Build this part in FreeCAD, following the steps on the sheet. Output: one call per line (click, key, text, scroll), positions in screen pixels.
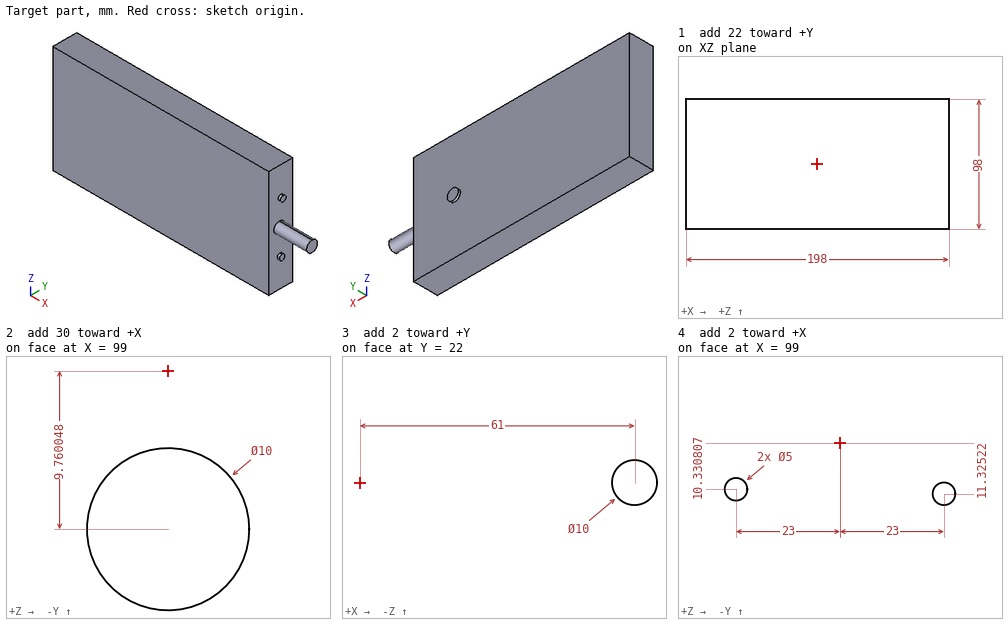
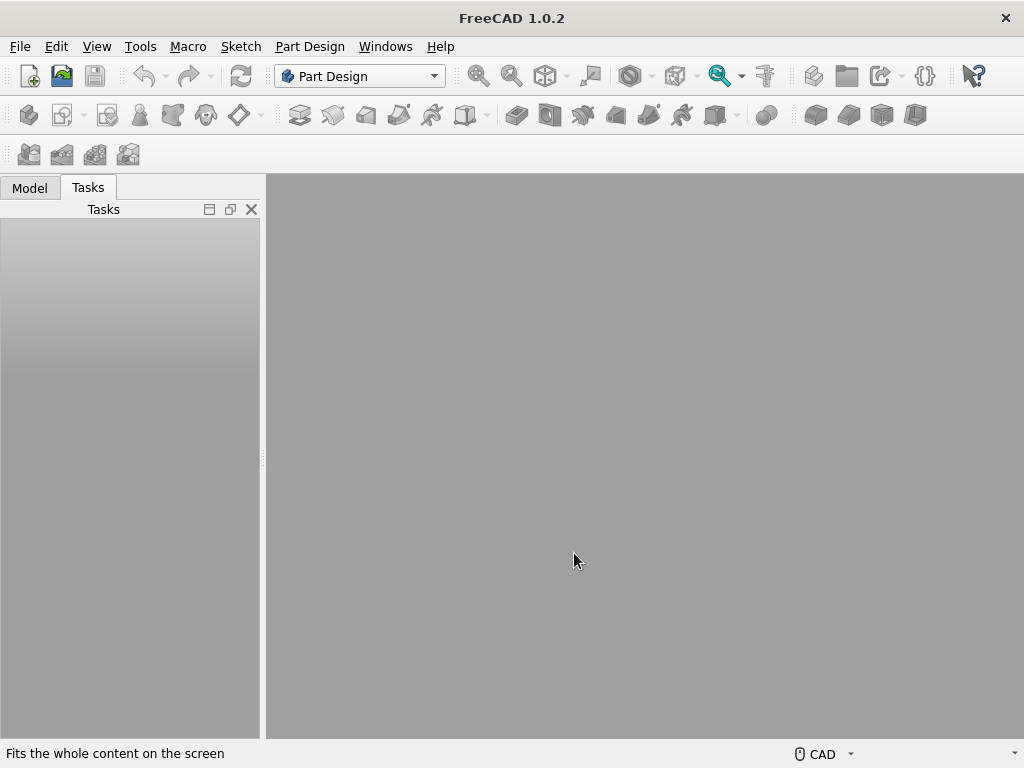
key(ctrl+n)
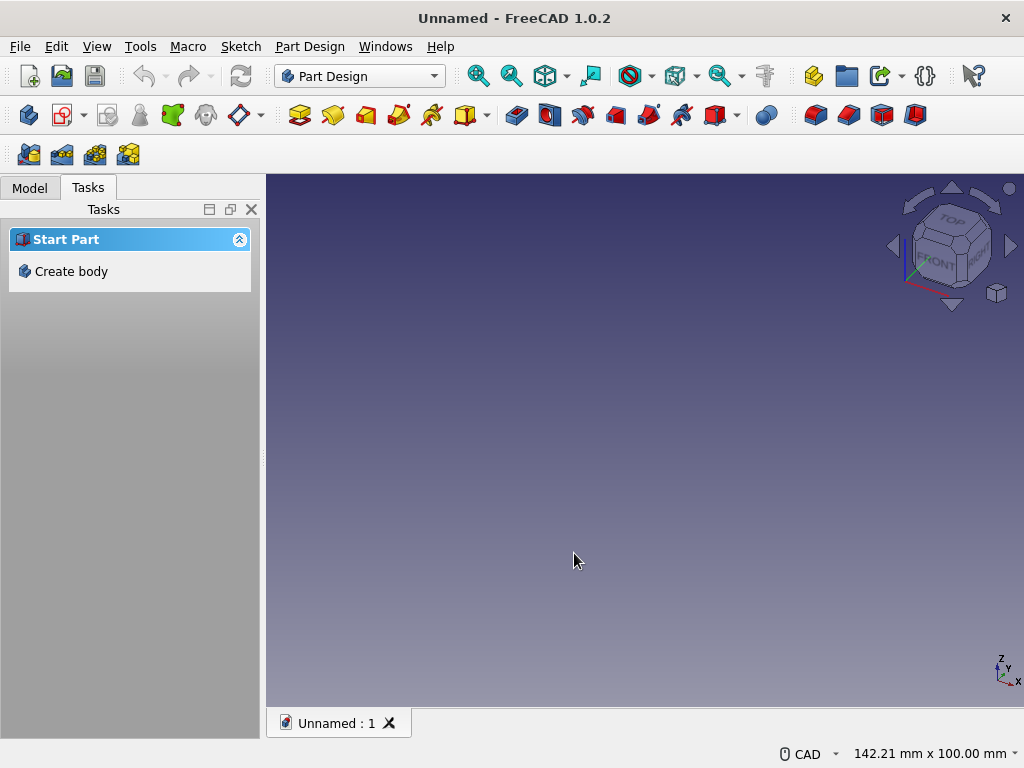
click(62, 116)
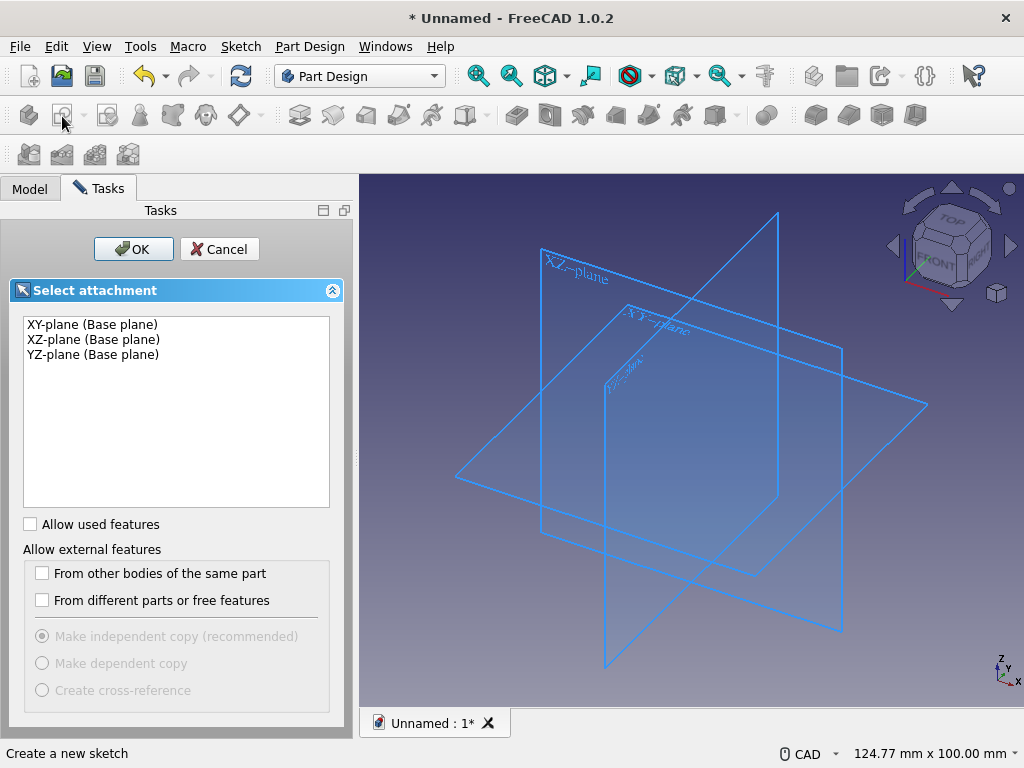
click(84, 340)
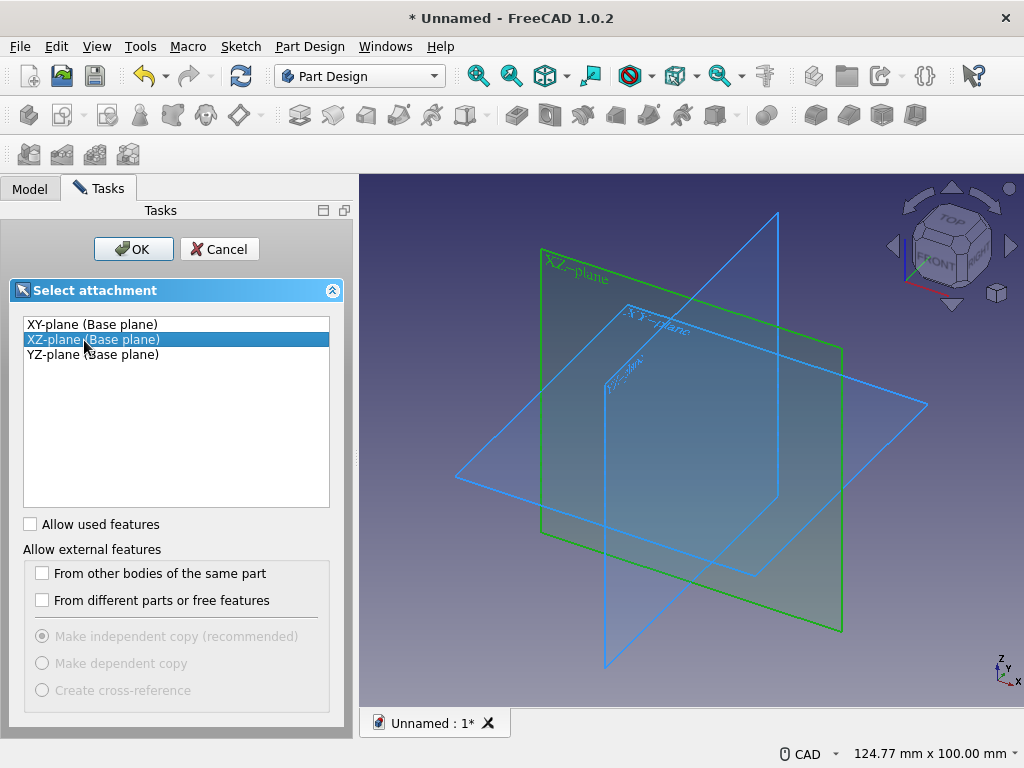
click(134, 249)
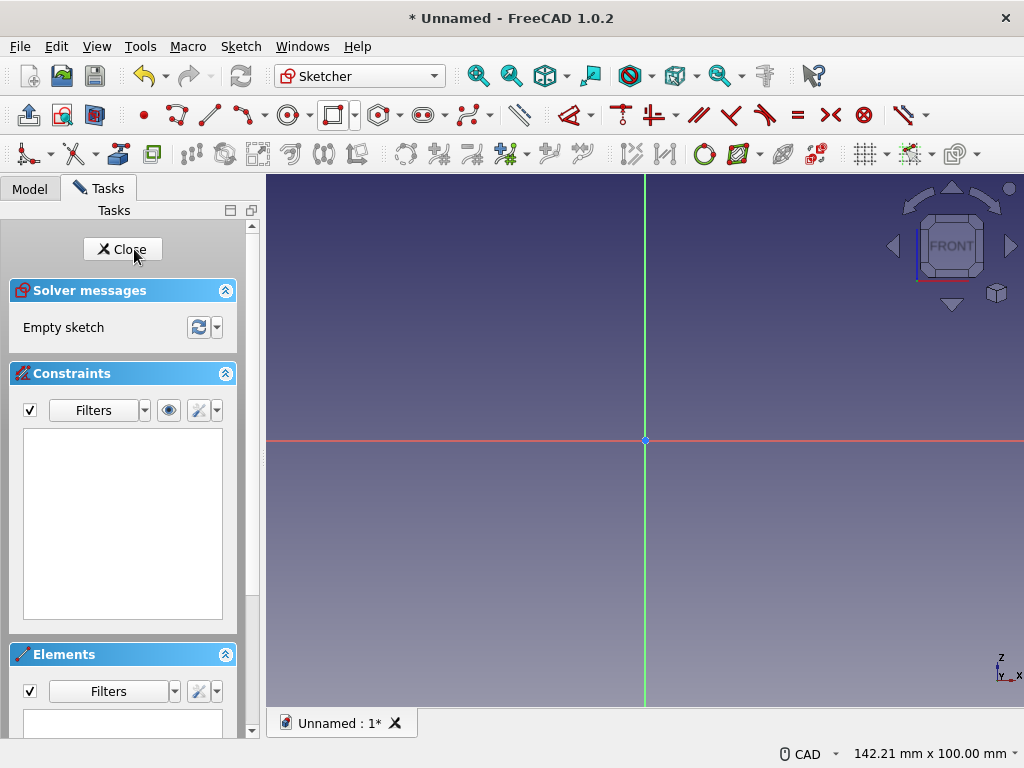
scroll(537, 440, down, 5)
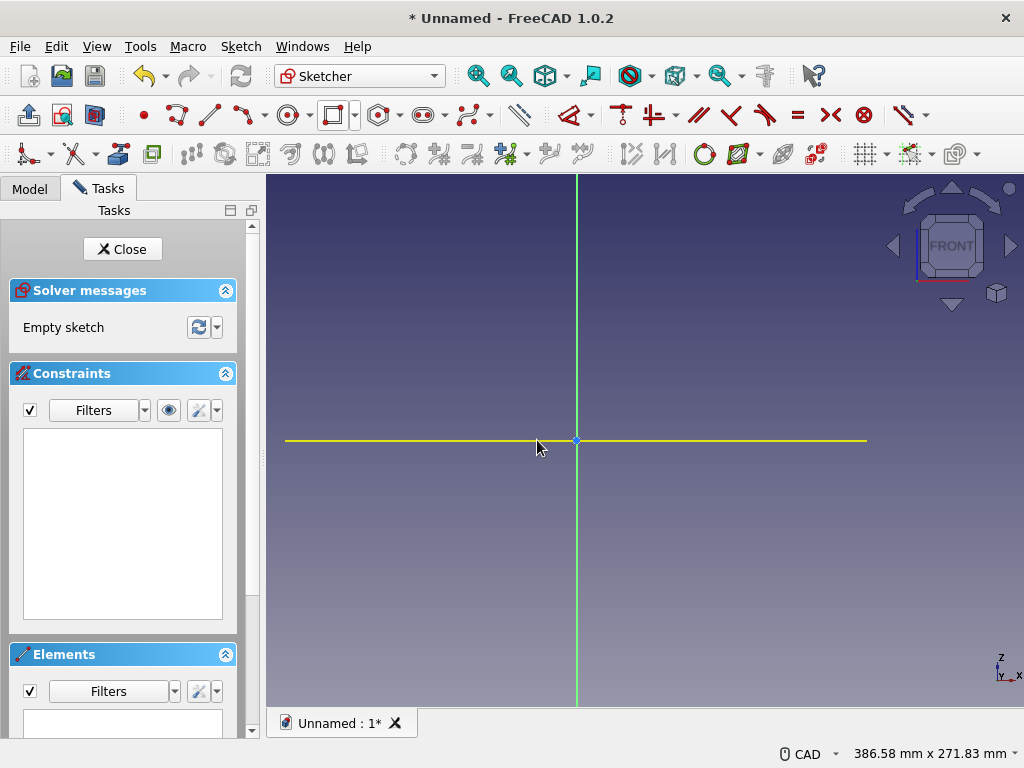
key(g)
key(v)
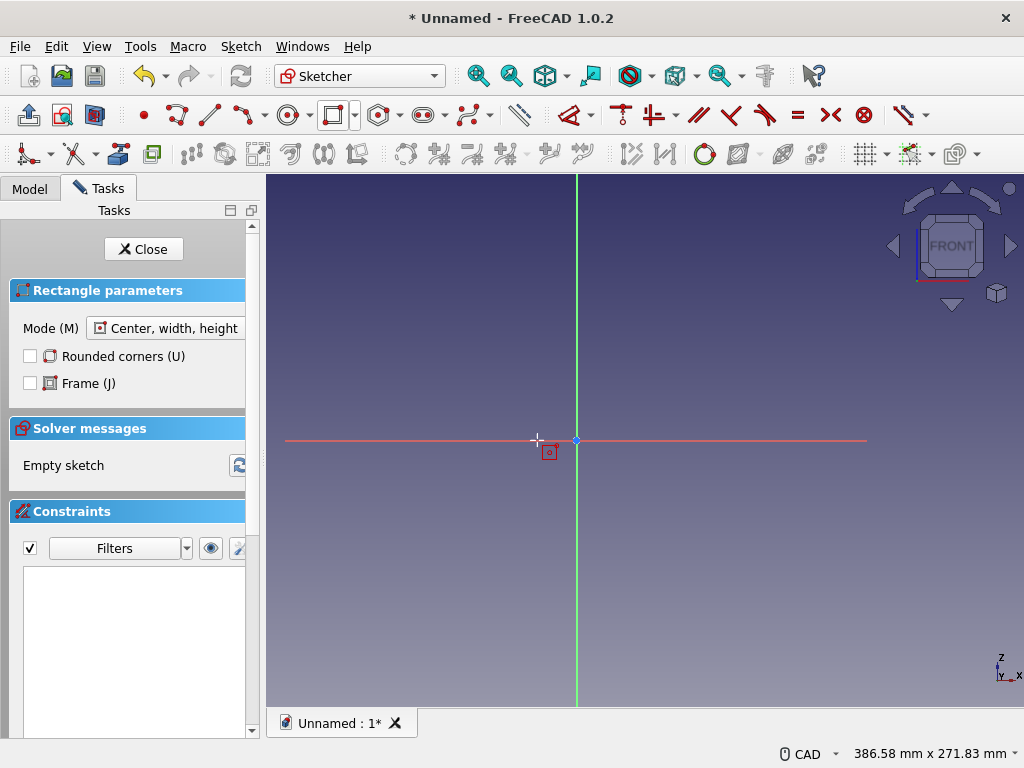
click(577, 440)
move(771, 344)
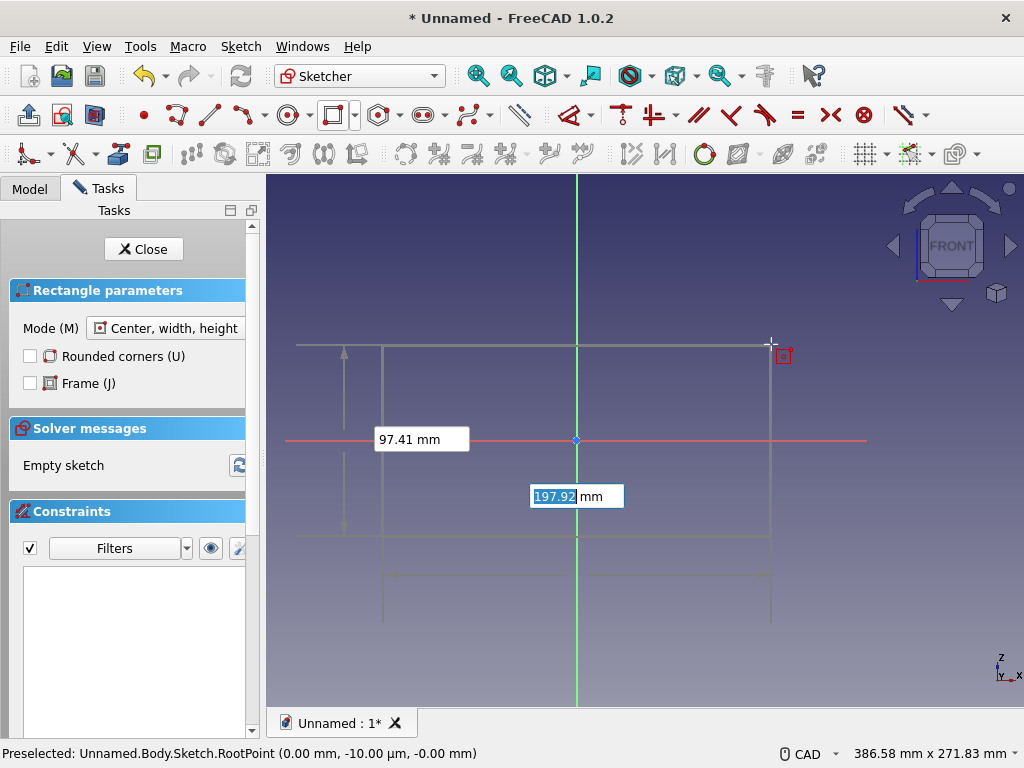
text(198)
key(Tab)
text(98)
key(Return)
key(Escape)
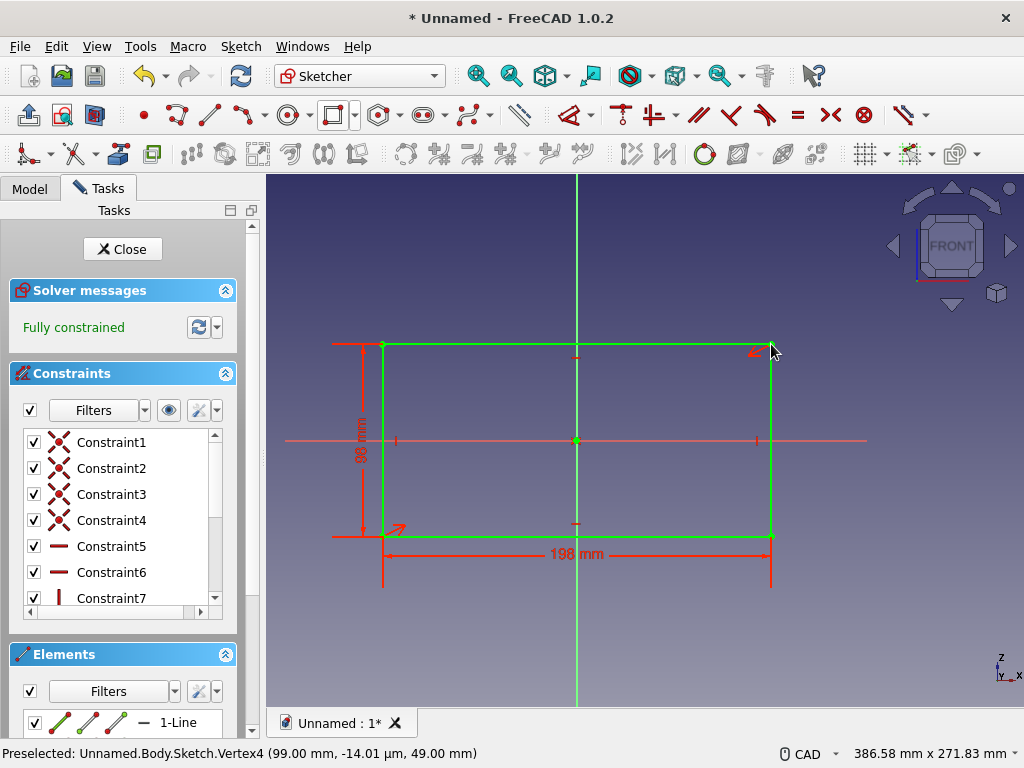
click(123, 249)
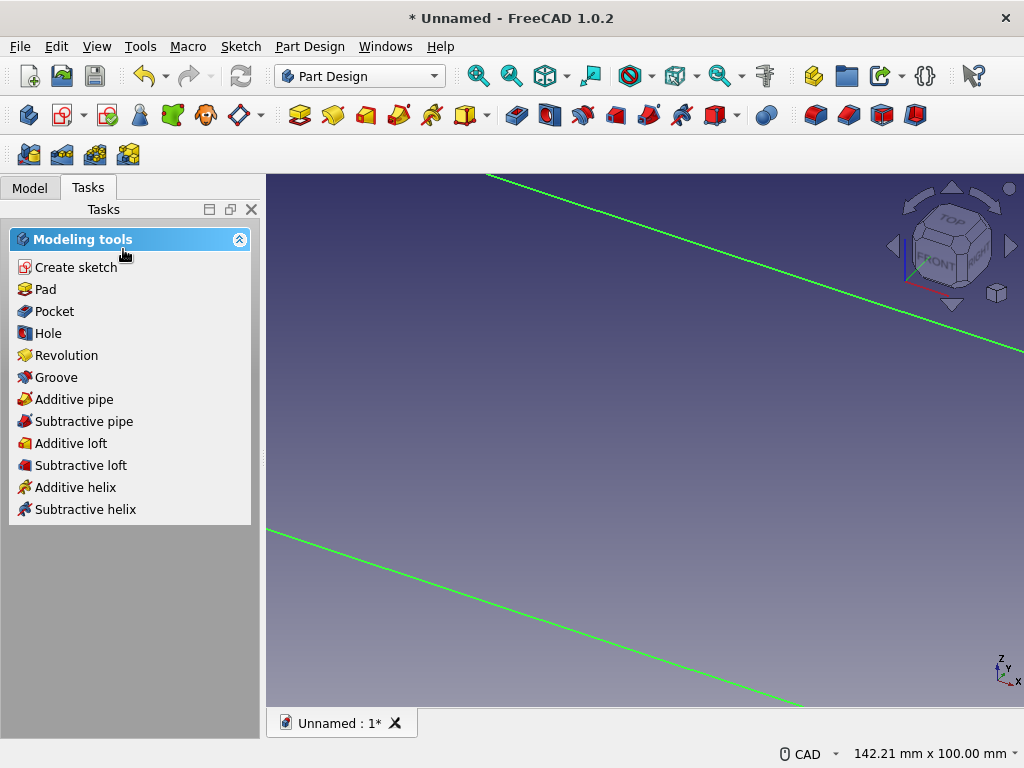
click(300, 116)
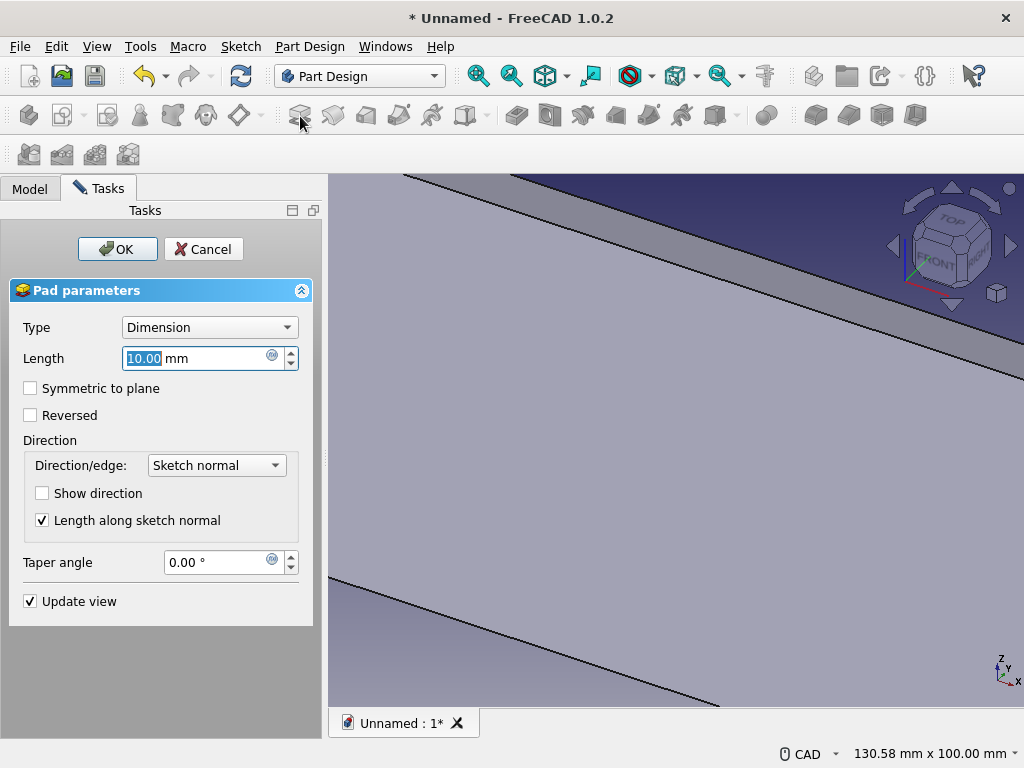
text(22)
key(Tab)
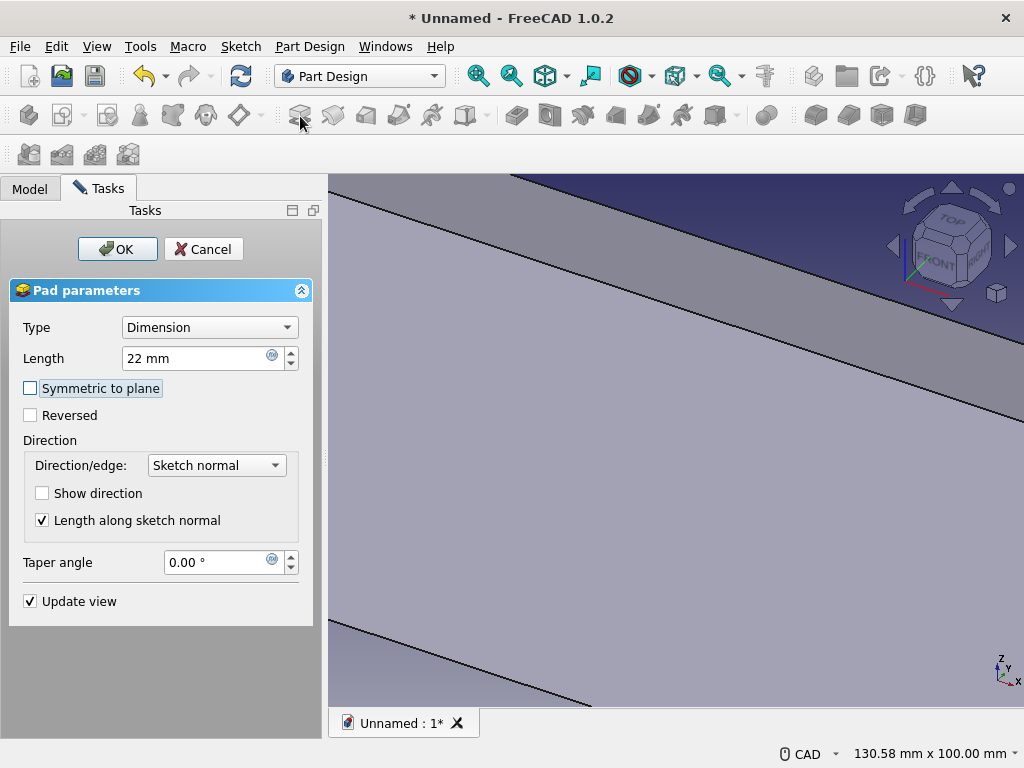
click(31, 415)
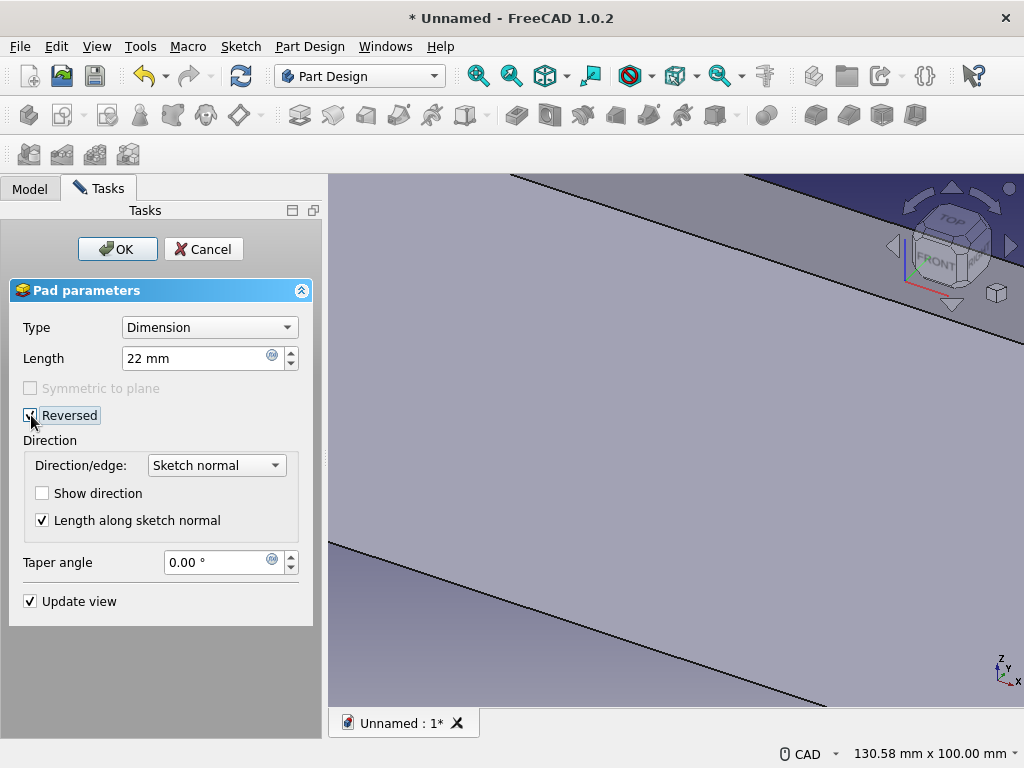
click(118, 249)